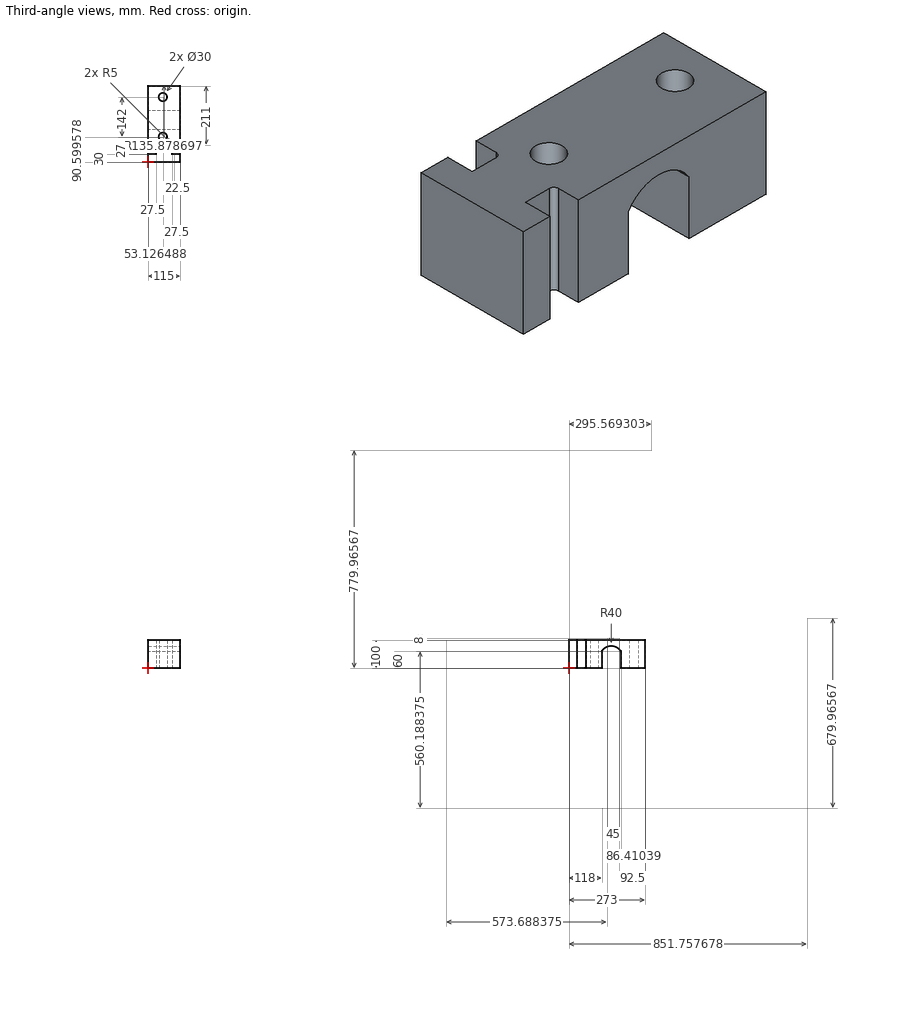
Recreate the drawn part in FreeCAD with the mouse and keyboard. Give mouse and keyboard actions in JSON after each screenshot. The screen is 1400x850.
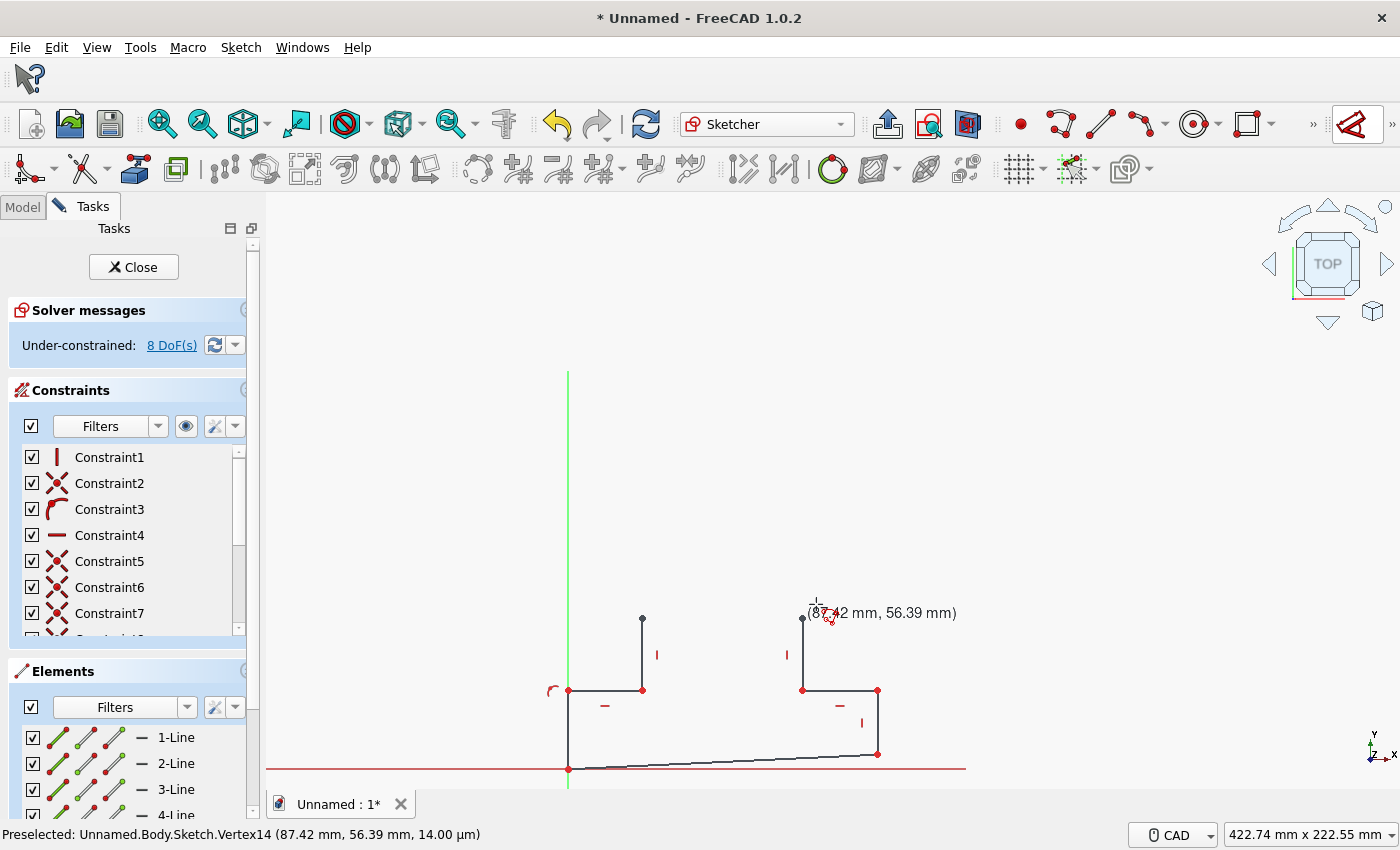
{"action": "left_click", "coordinate": [816, 603]}
{"action": "left_click", "coordinate": [877, 603]}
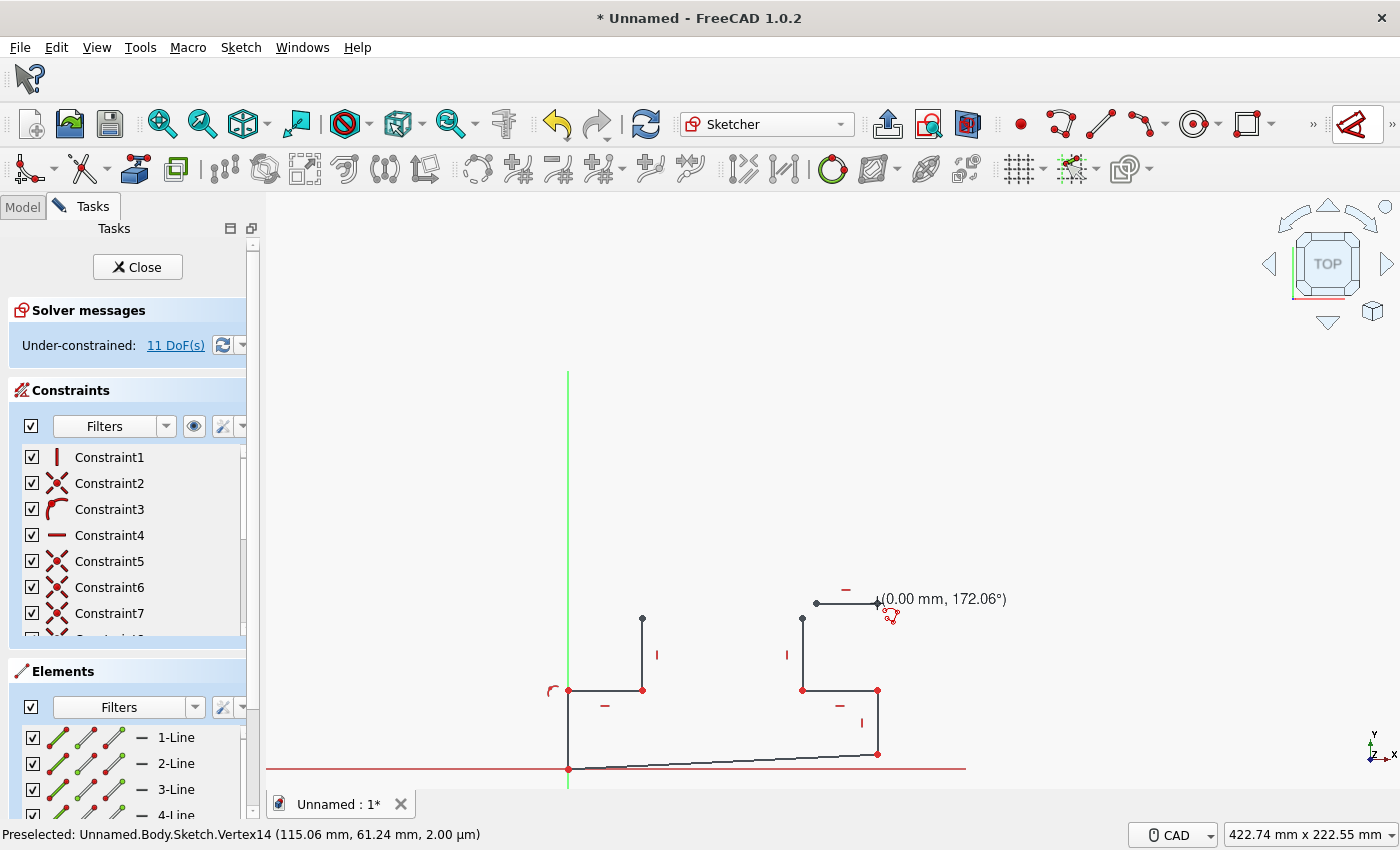
{"action": "scroll", "coordinate": [815, 618], "scroll_direction": "down", "scroll_amount": 3}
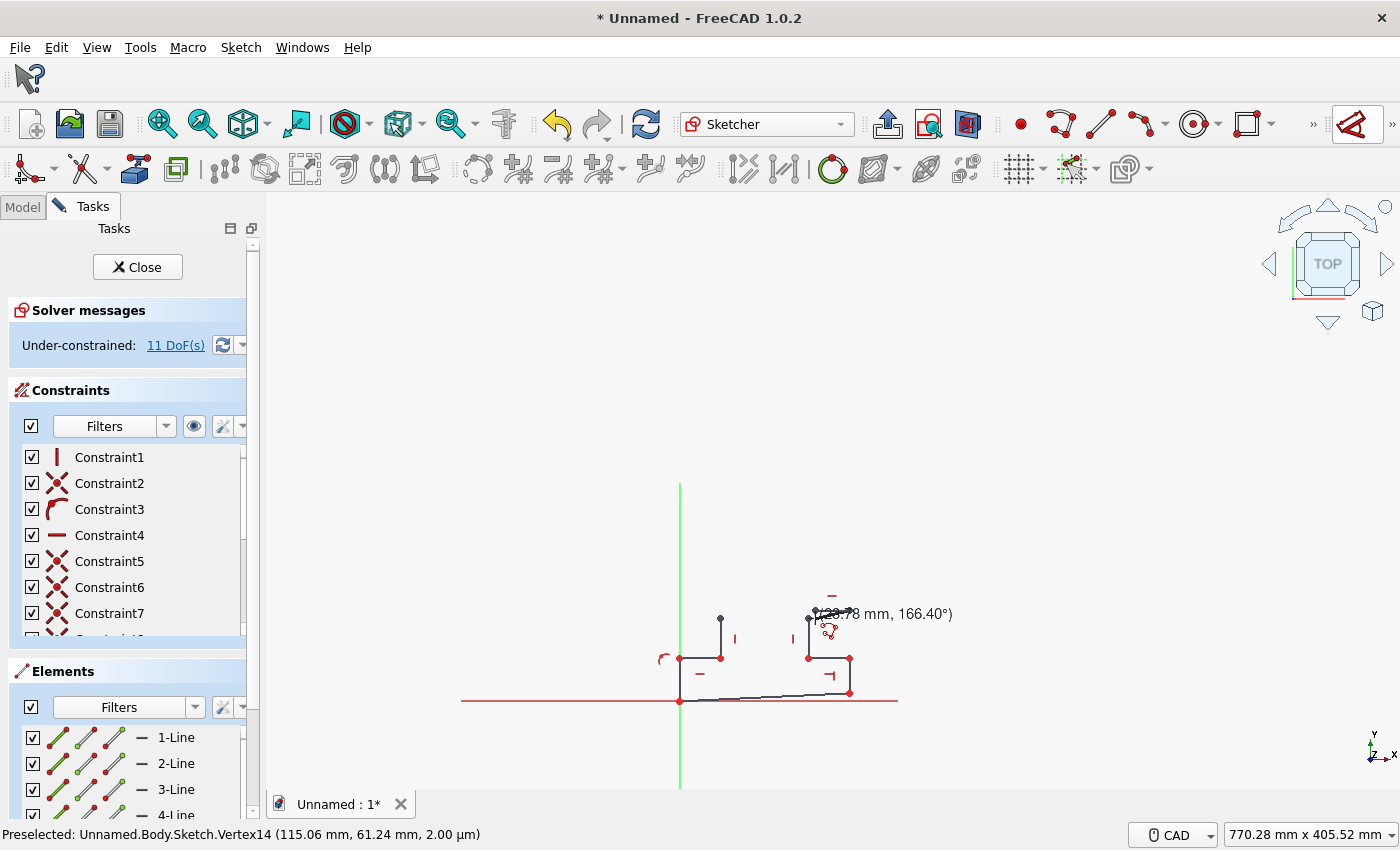
{"action": "left_click", "coordinate": [849, 299]}
{"action": "right_click", "coordinate": [849, 299]}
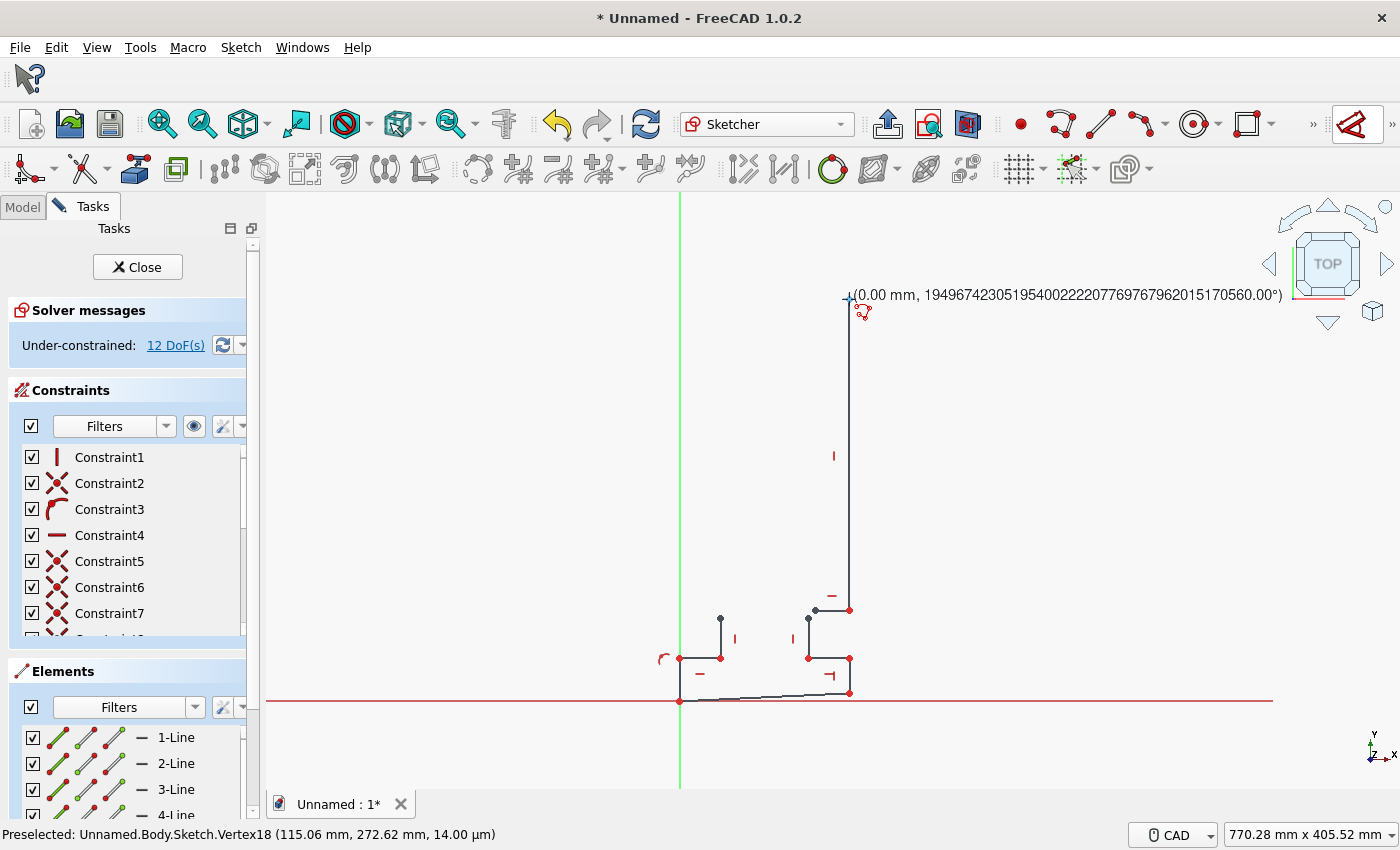
{"action": "left_click", "coordinate": [680, 299]}
{"action": "left_click", "coordinate": [689, 610]}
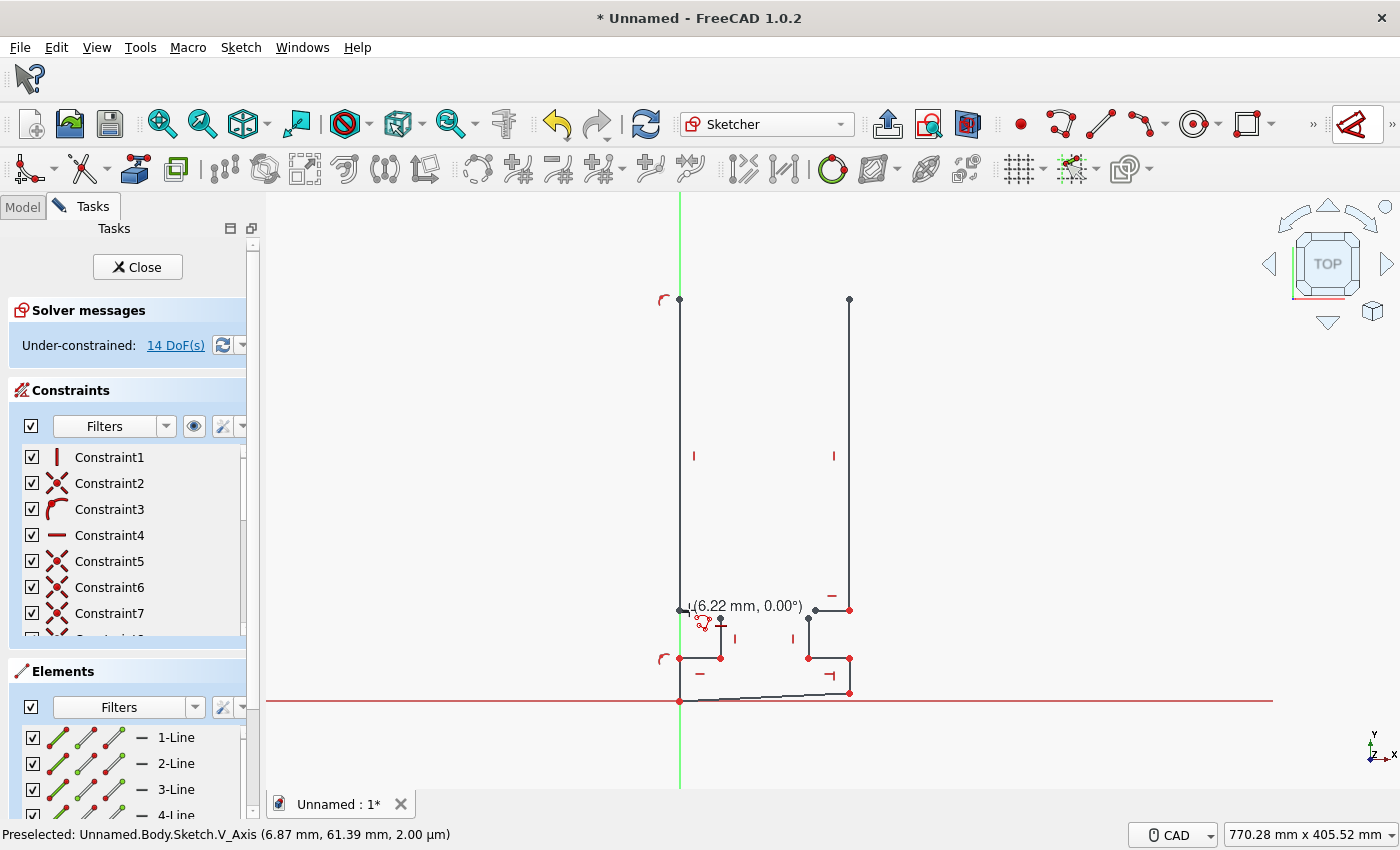
{"action": "scroll", "coordinate": [713, 610], "scroll_direction": "up", "scroll_amount": 3}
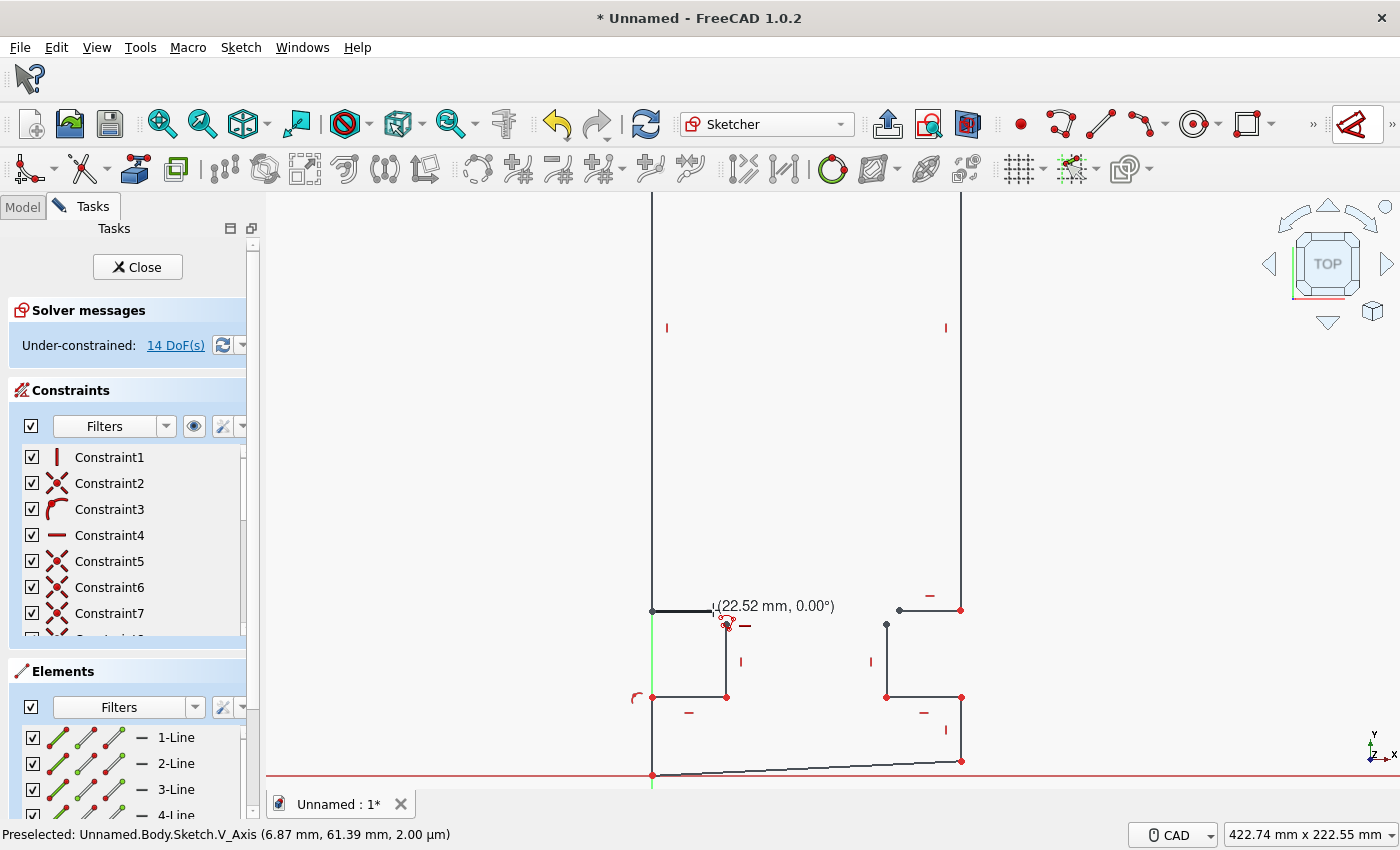
{"action": "left_click", "coordinate": [713, 609]}
{"action": "right_click", "coordinate": [713, 609]}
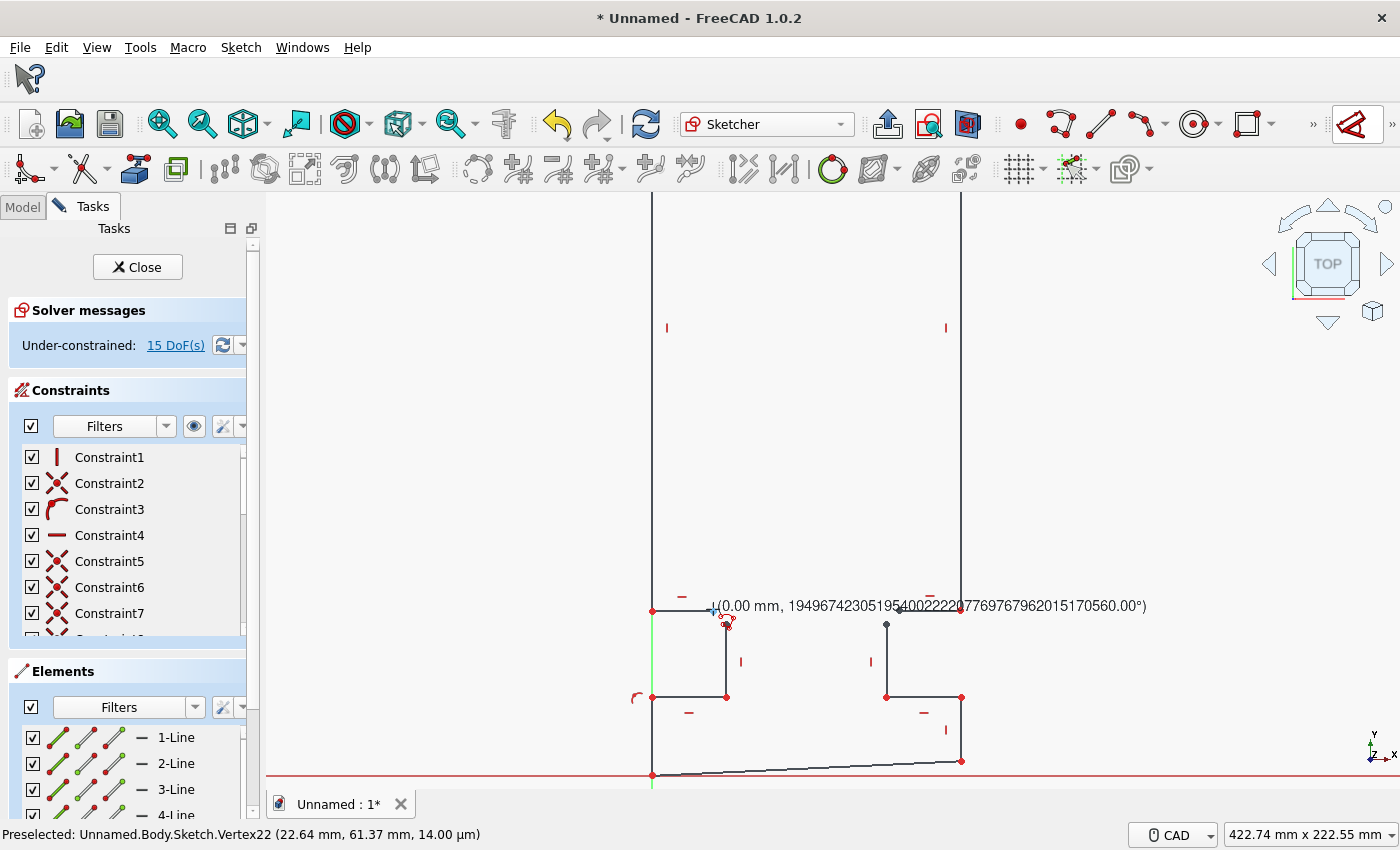
{"action": "key", "text": "g 3 a"}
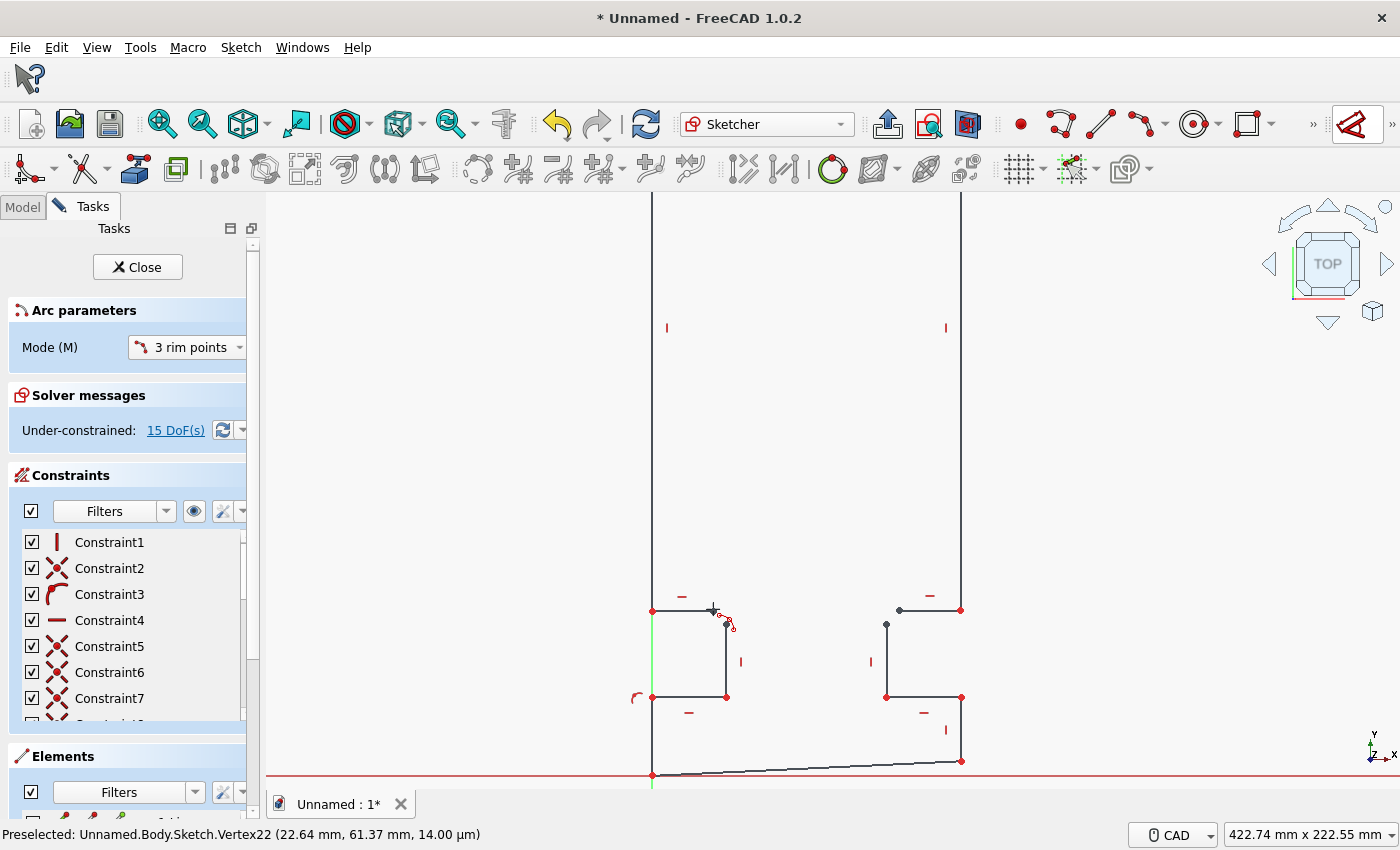
{"action": "left_click", "coordinate": [887, 625]}
{"action": "left_click", "coordinate": [900, 611]}